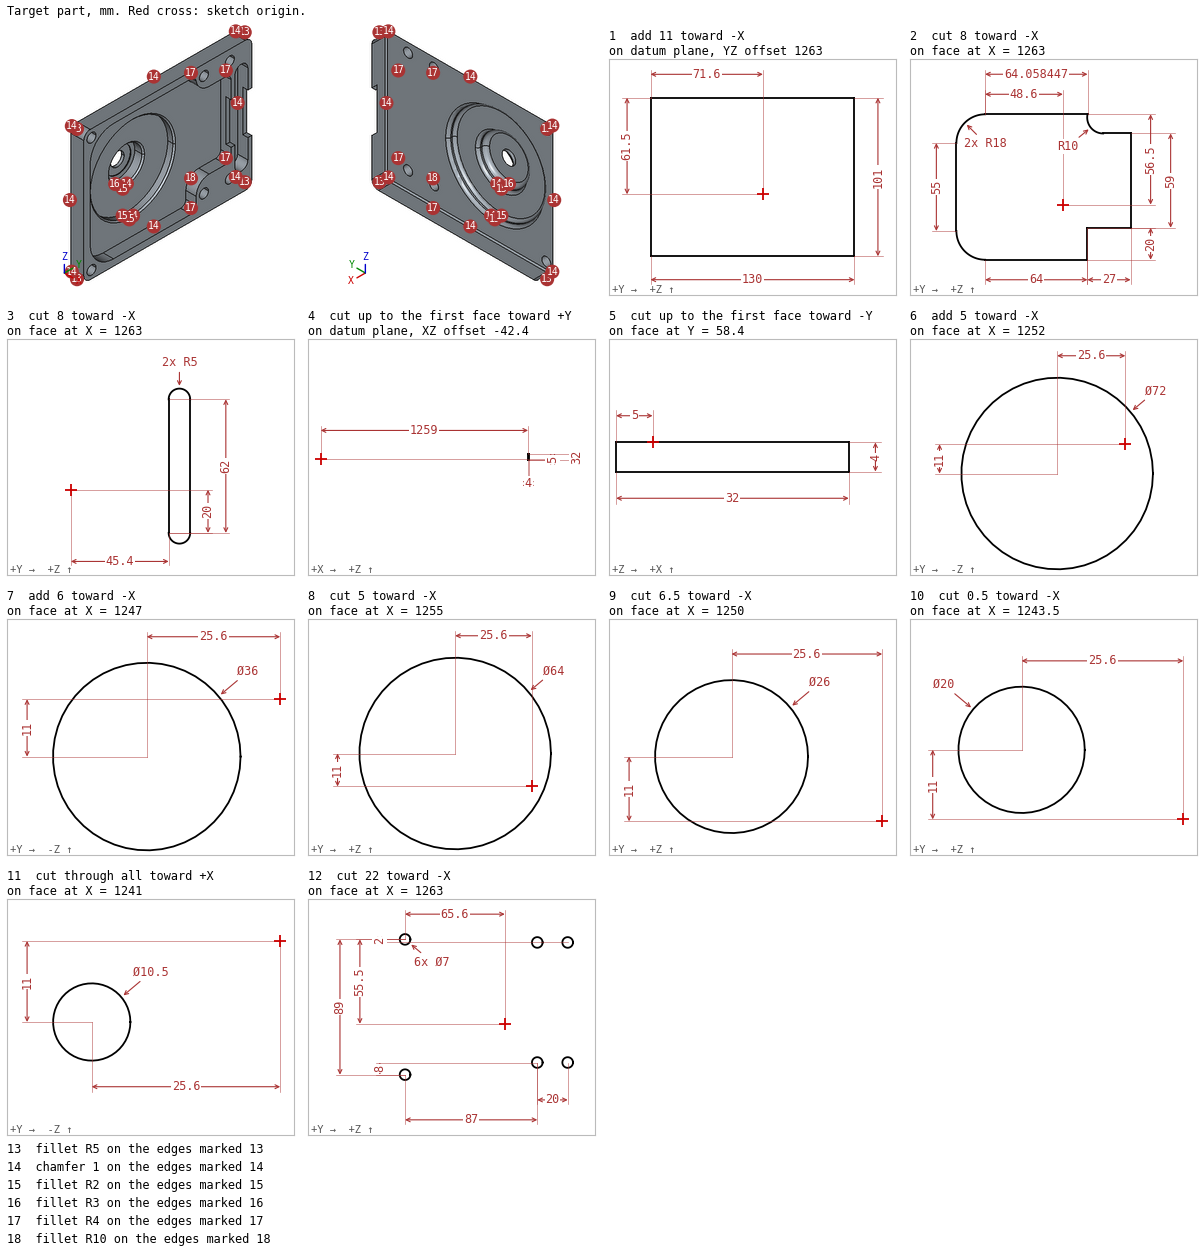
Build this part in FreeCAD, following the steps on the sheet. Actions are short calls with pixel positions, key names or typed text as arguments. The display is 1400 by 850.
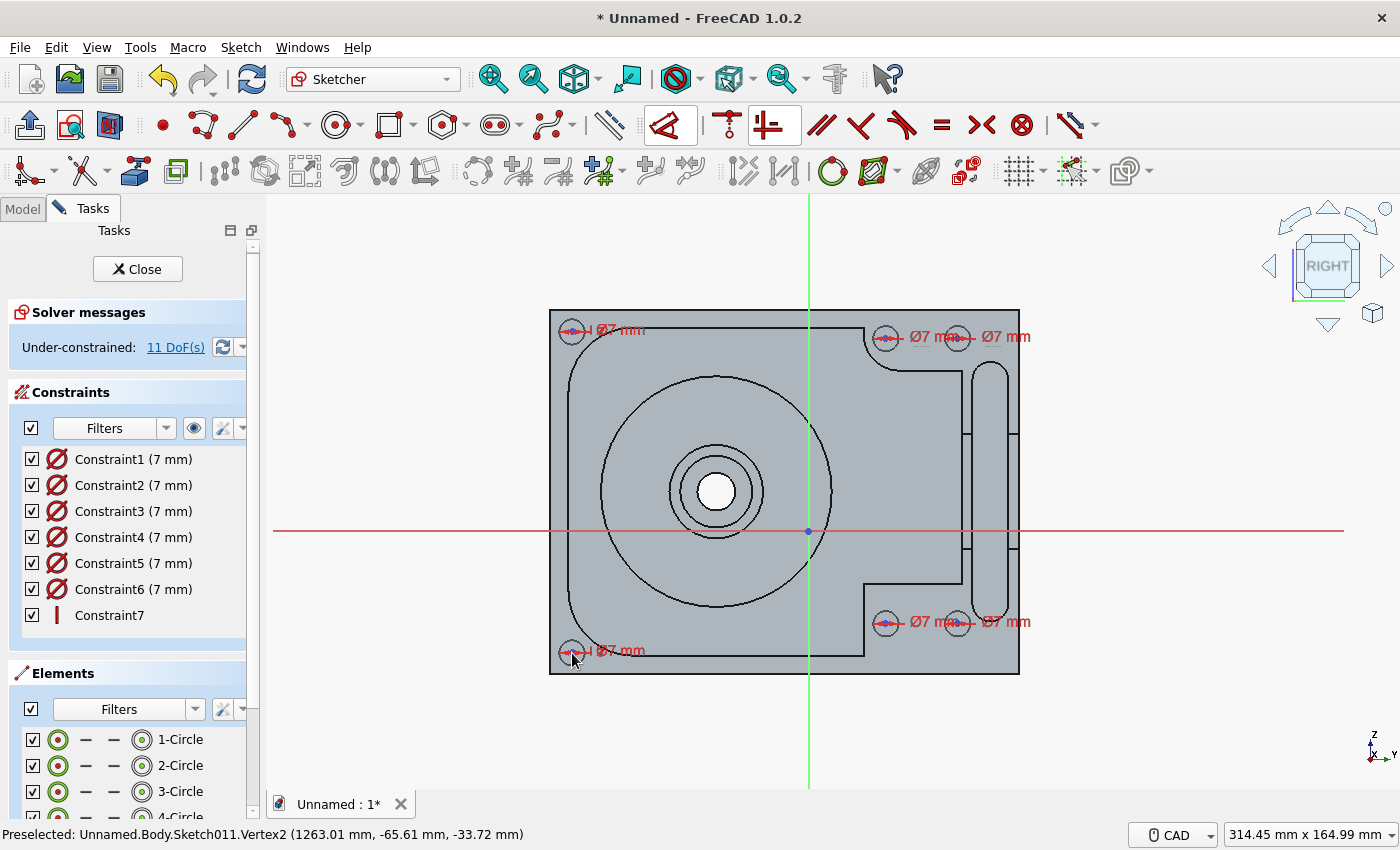
click(886, 624)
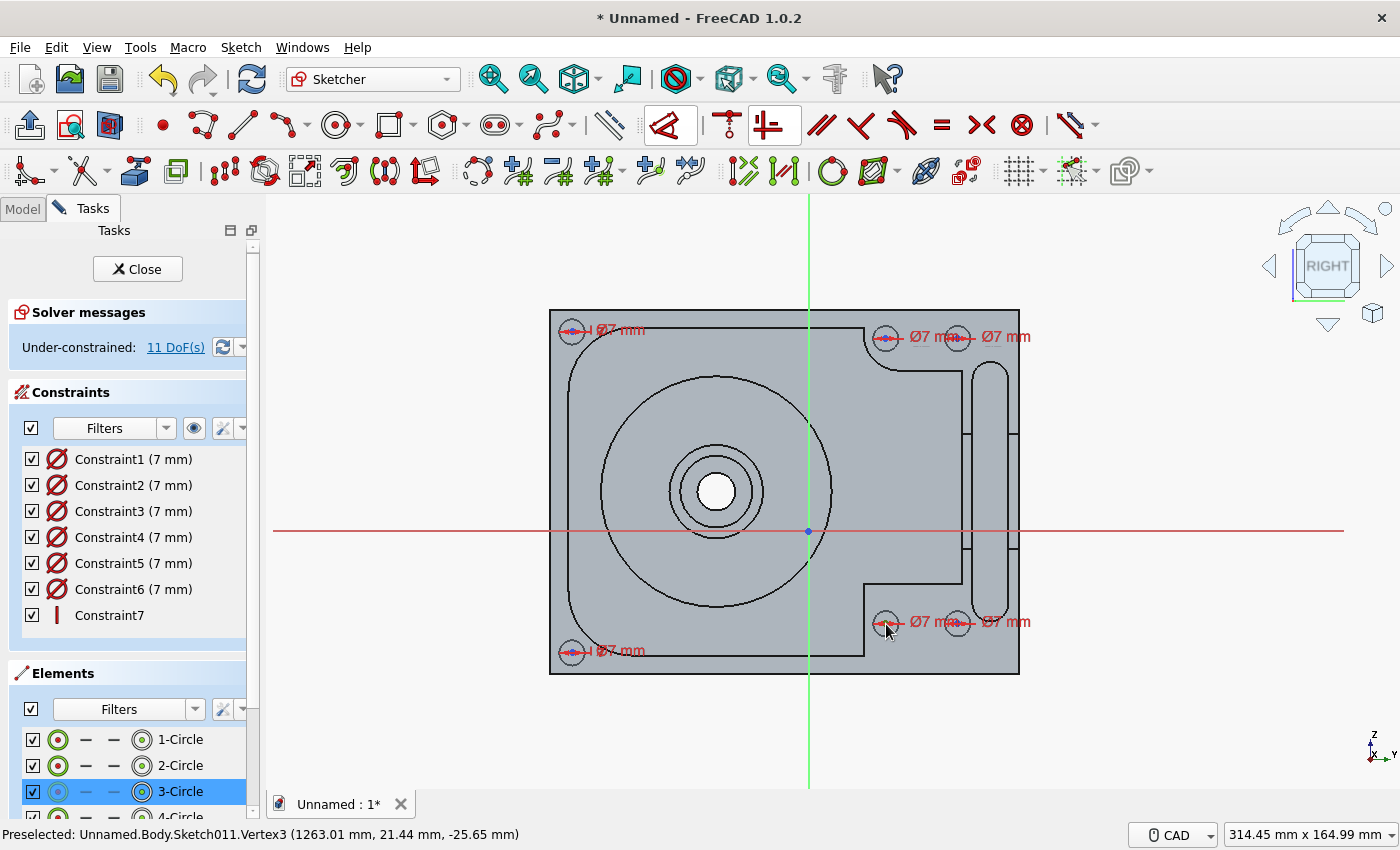
click(958, 624)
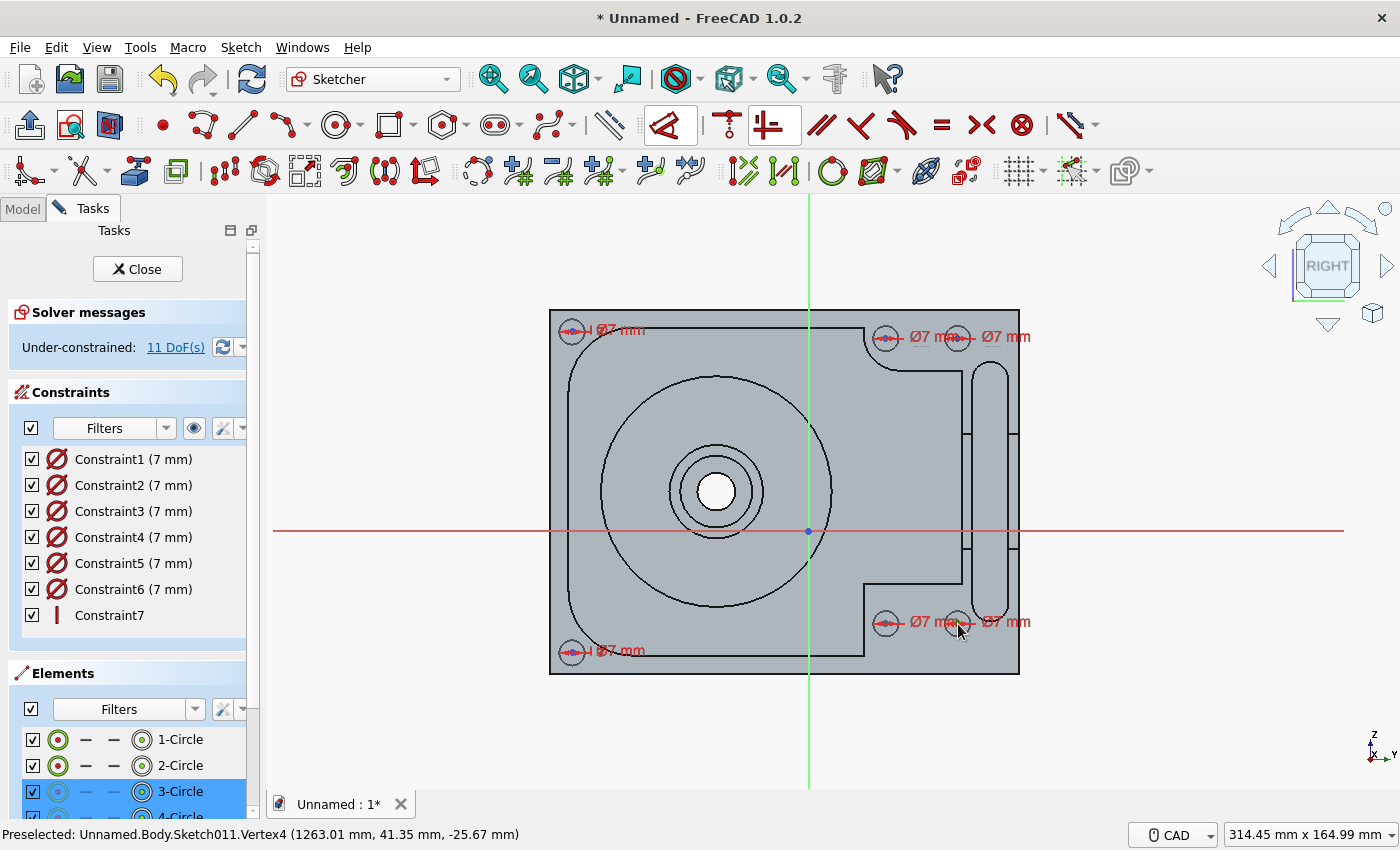
key(h)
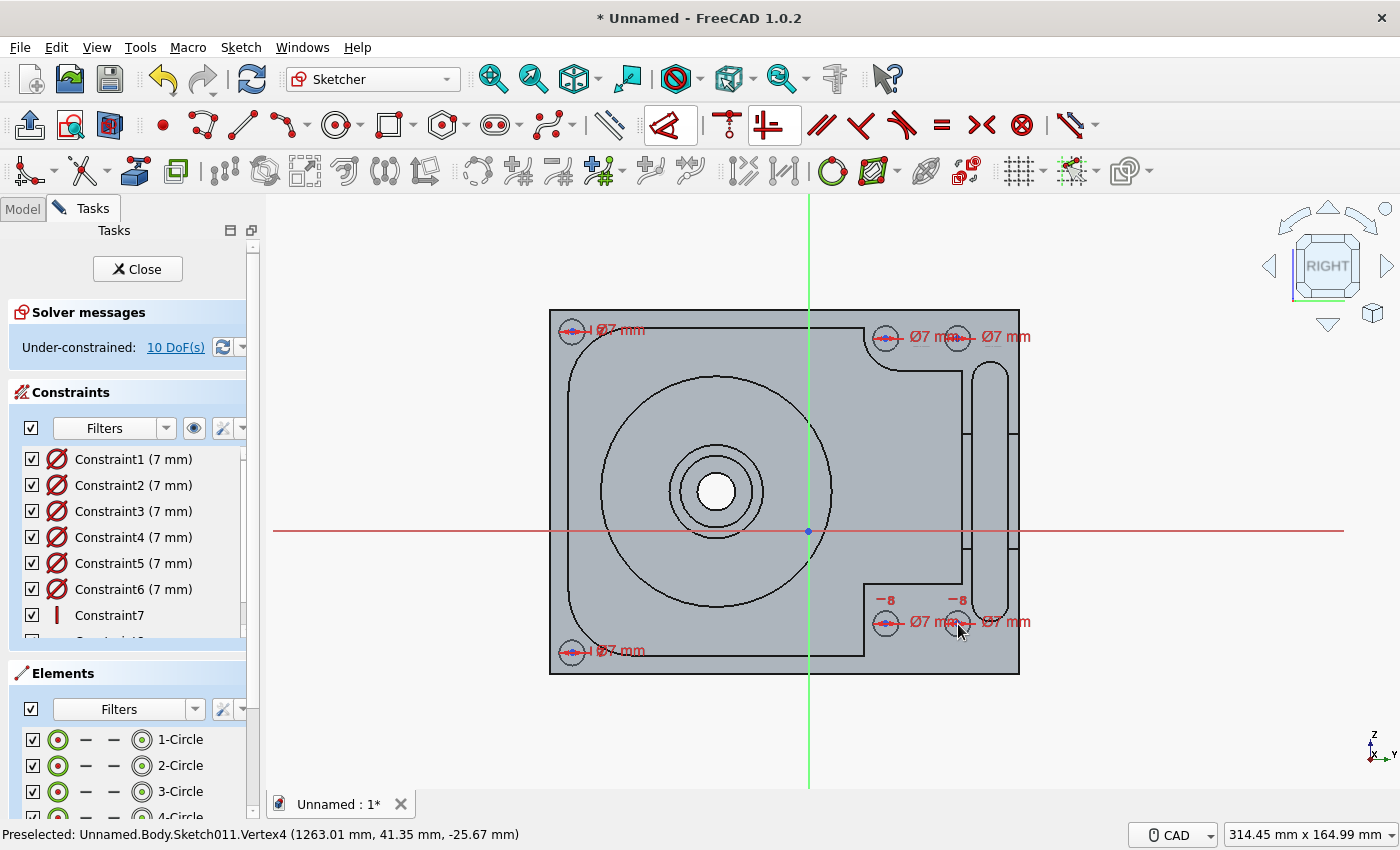
click(958, 624)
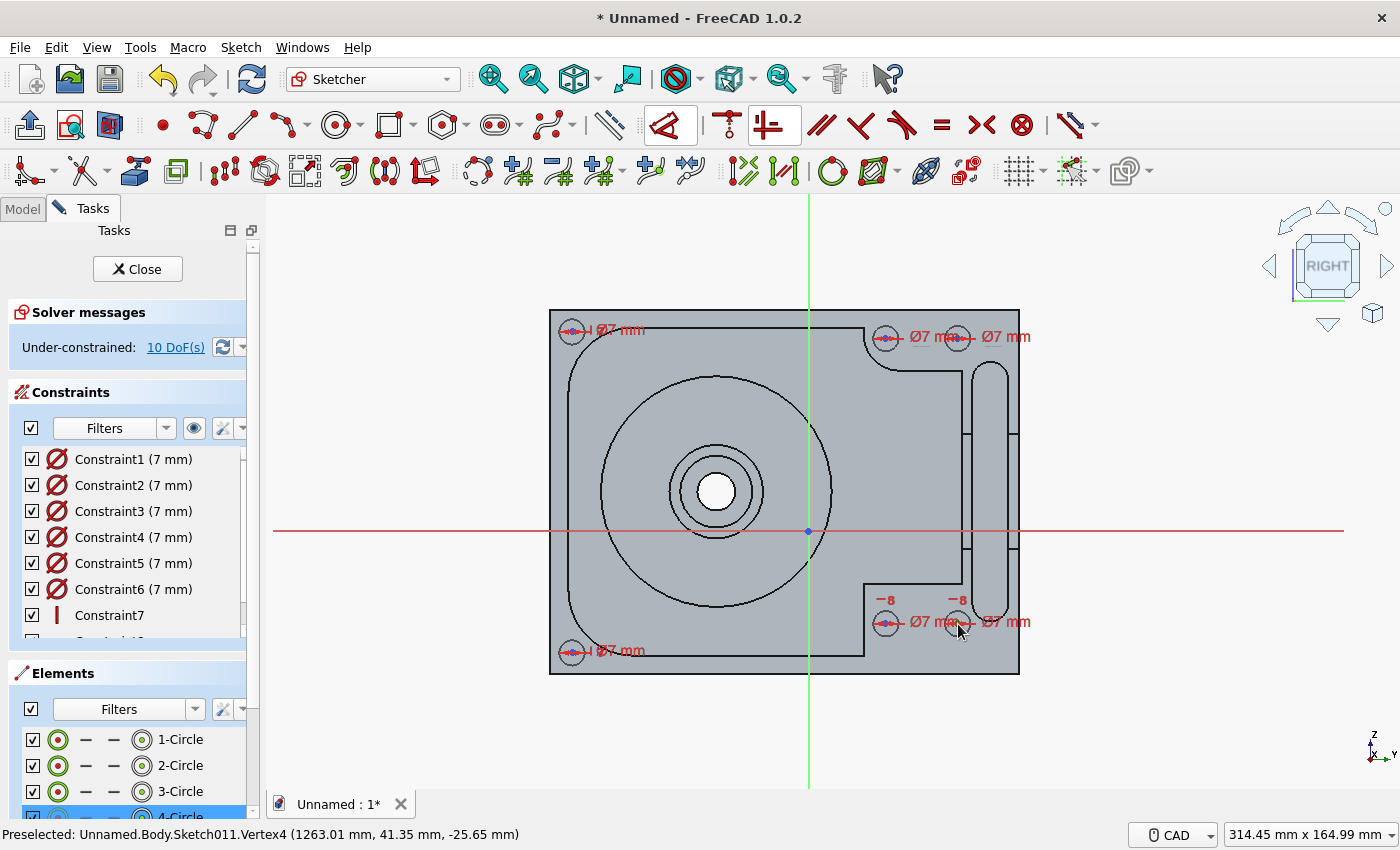
click(958, 339)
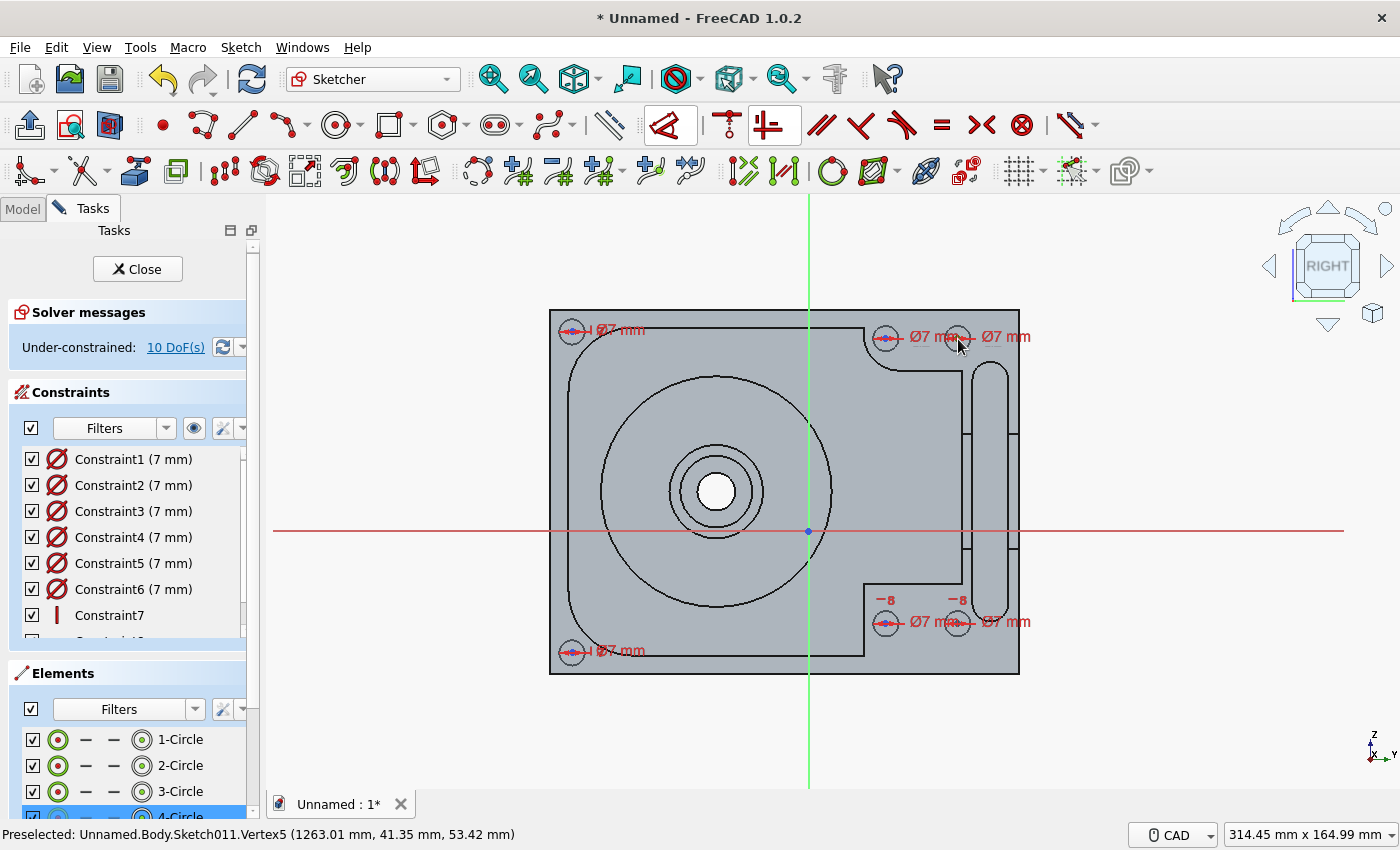
key(v)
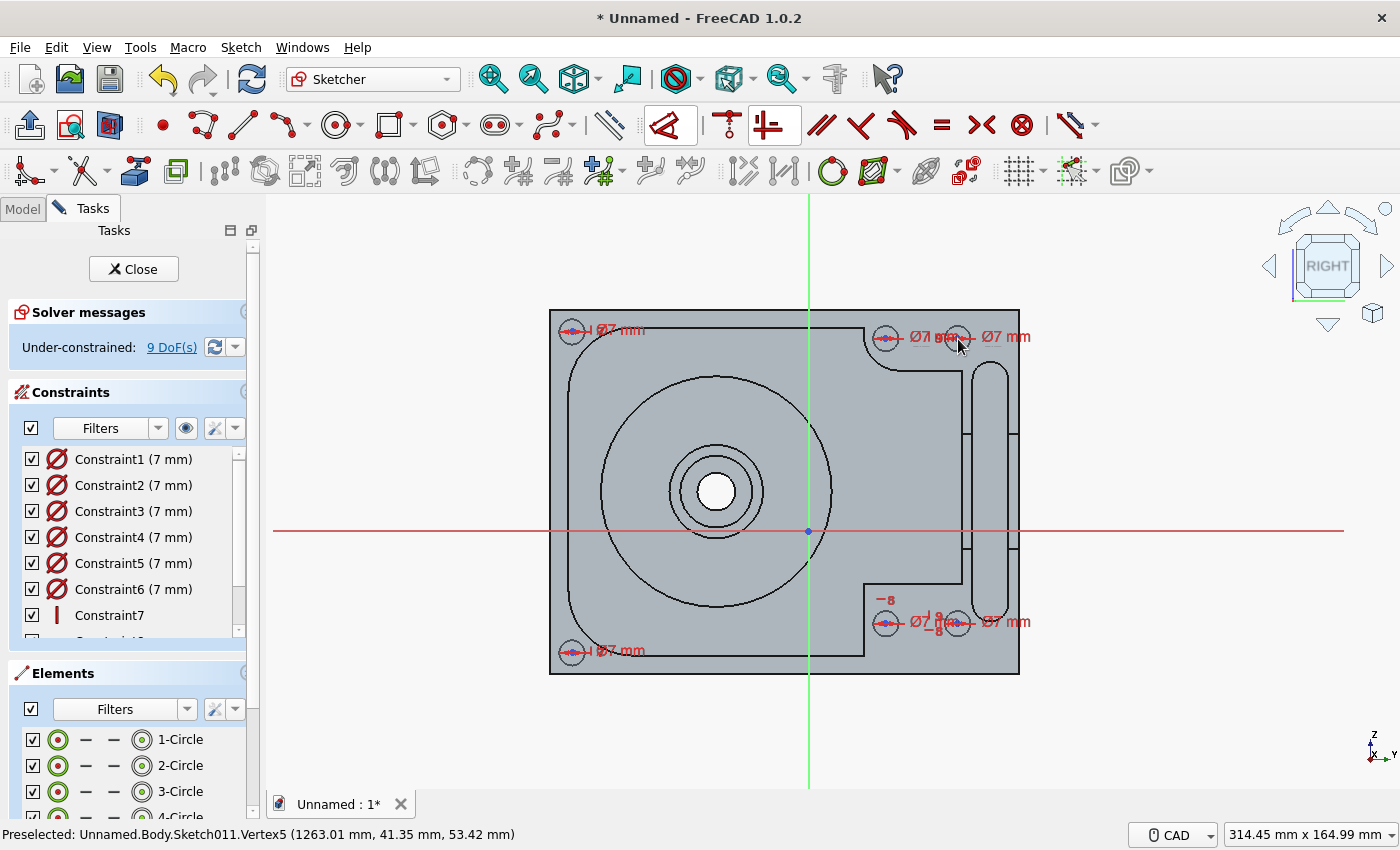
click(886, 624)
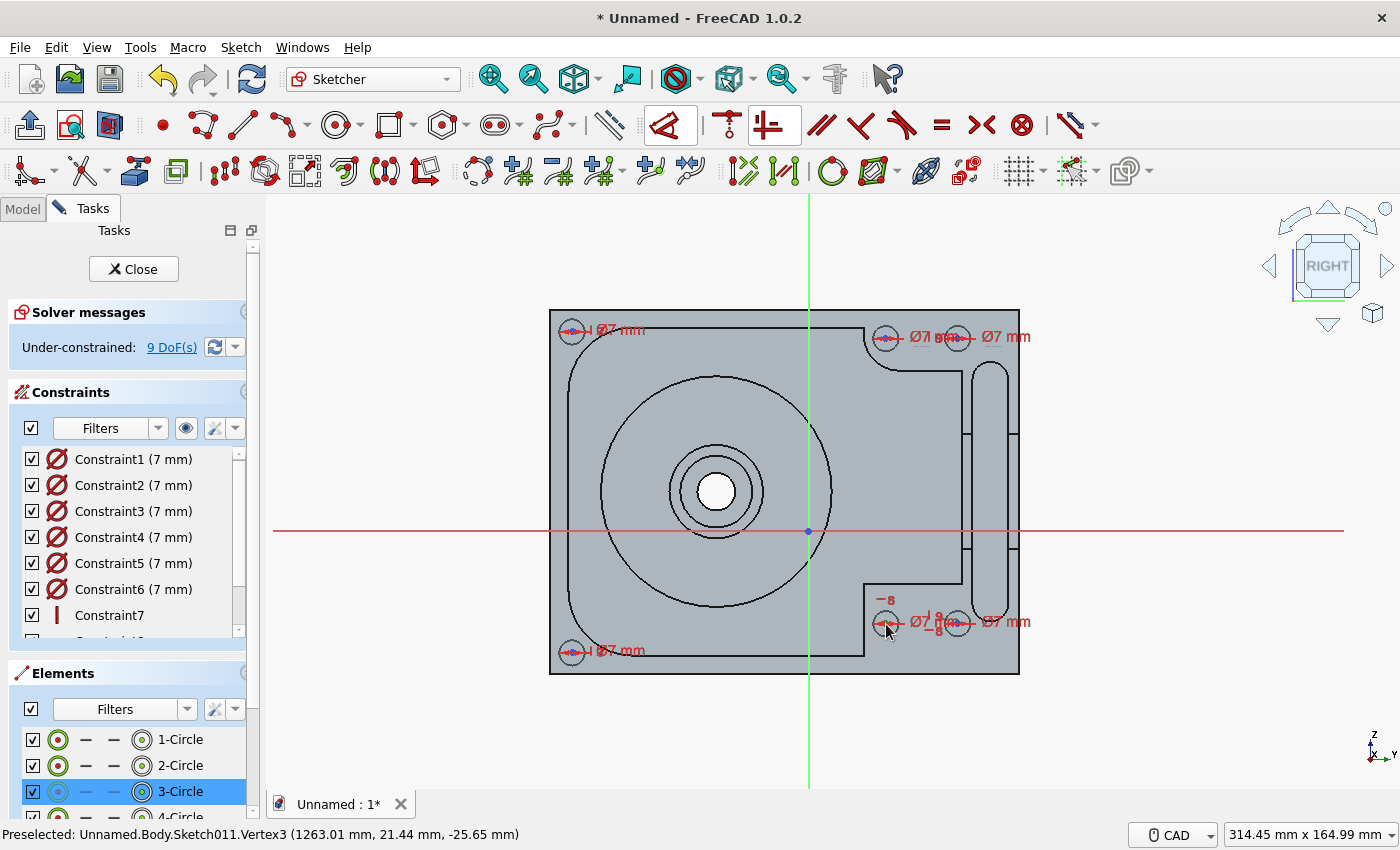
click(886, 339)